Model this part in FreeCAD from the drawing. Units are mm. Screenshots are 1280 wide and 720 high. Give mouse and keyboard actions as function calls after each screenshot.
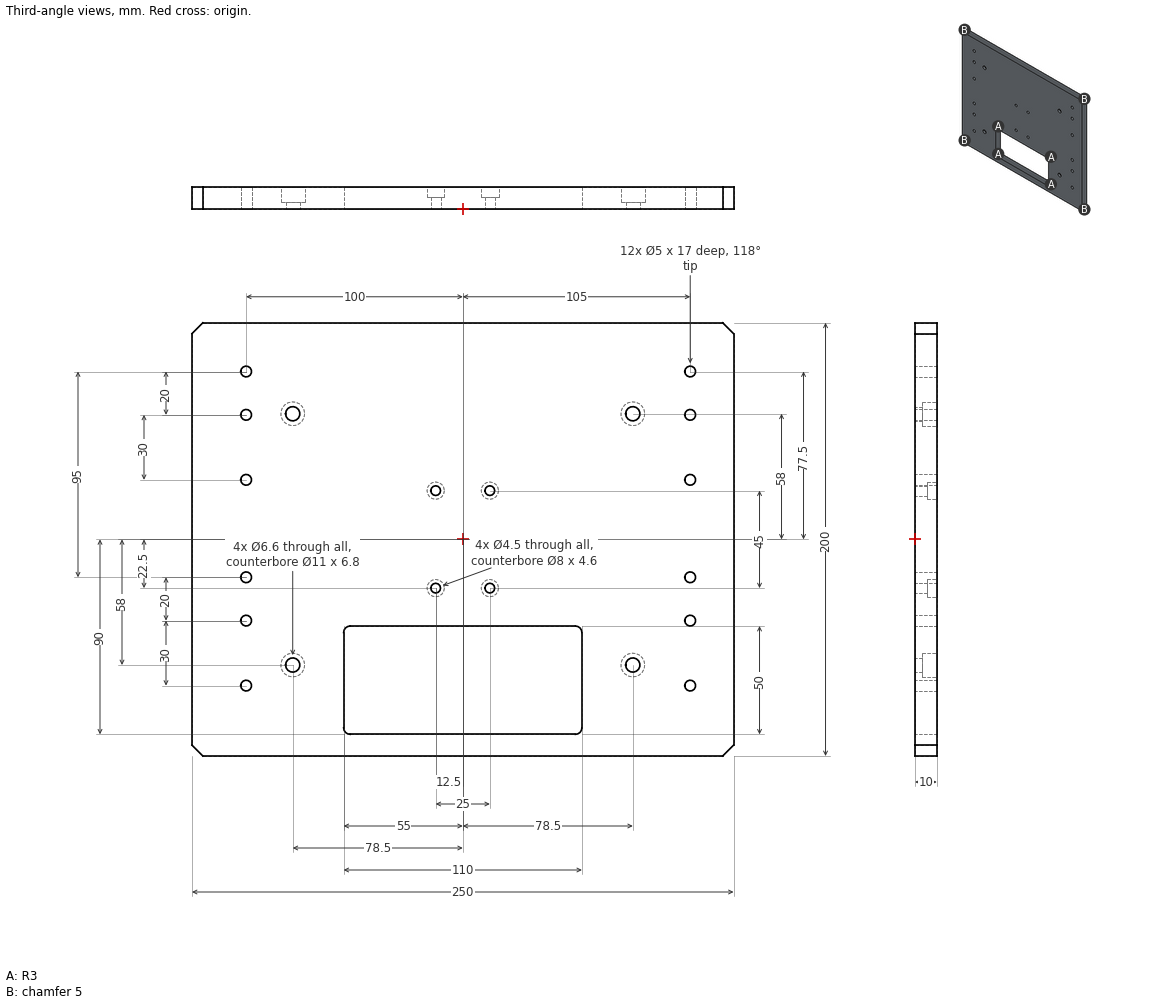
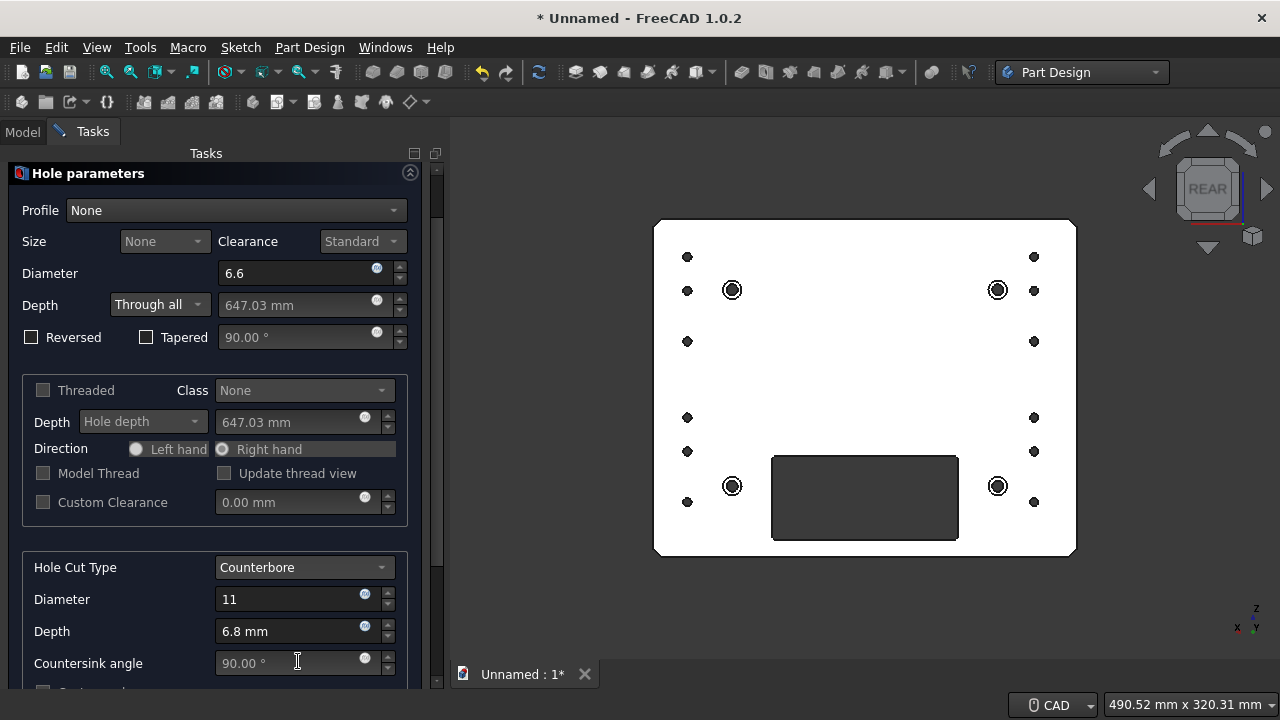
scroll(437, 426, up, 2)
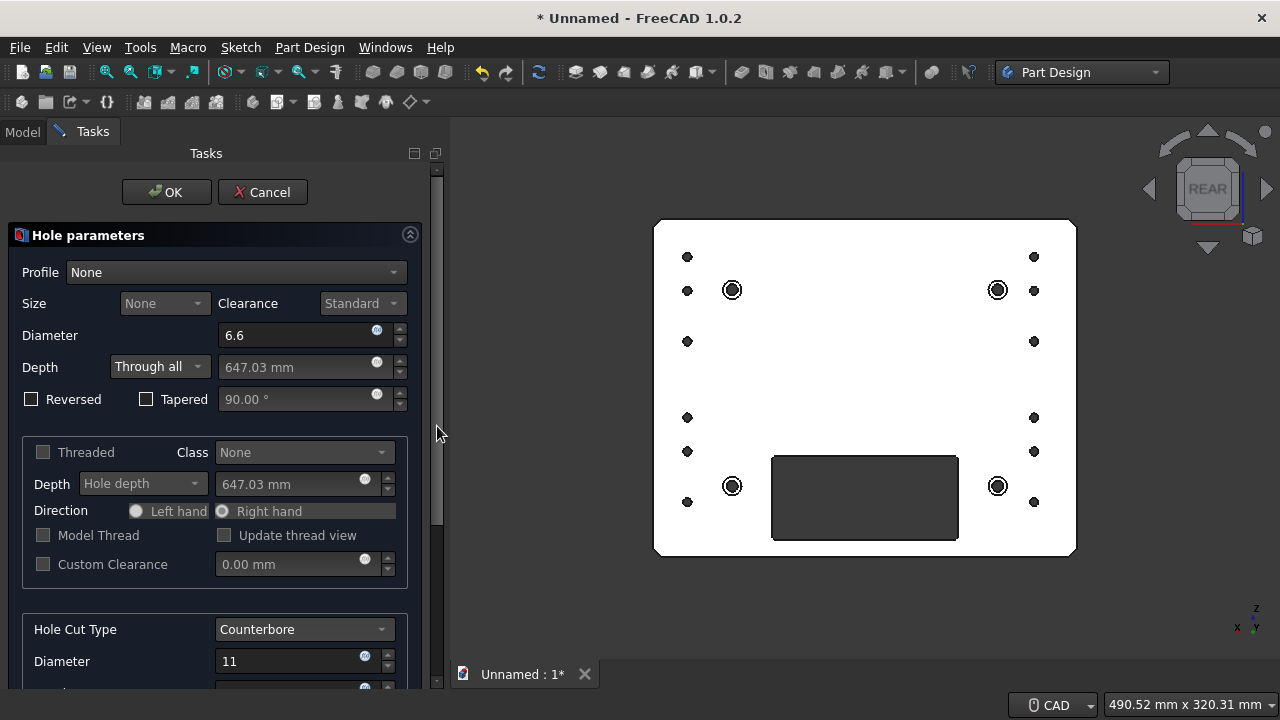
click(167, 192)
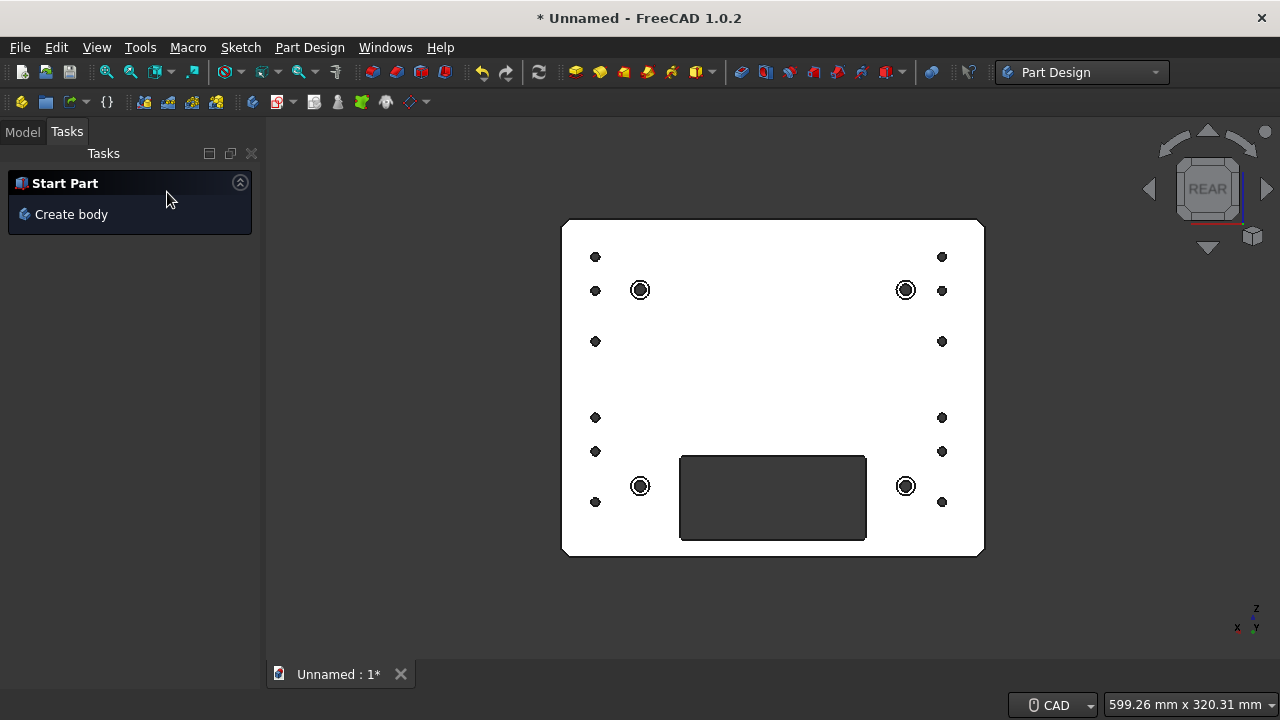
click(773, 339)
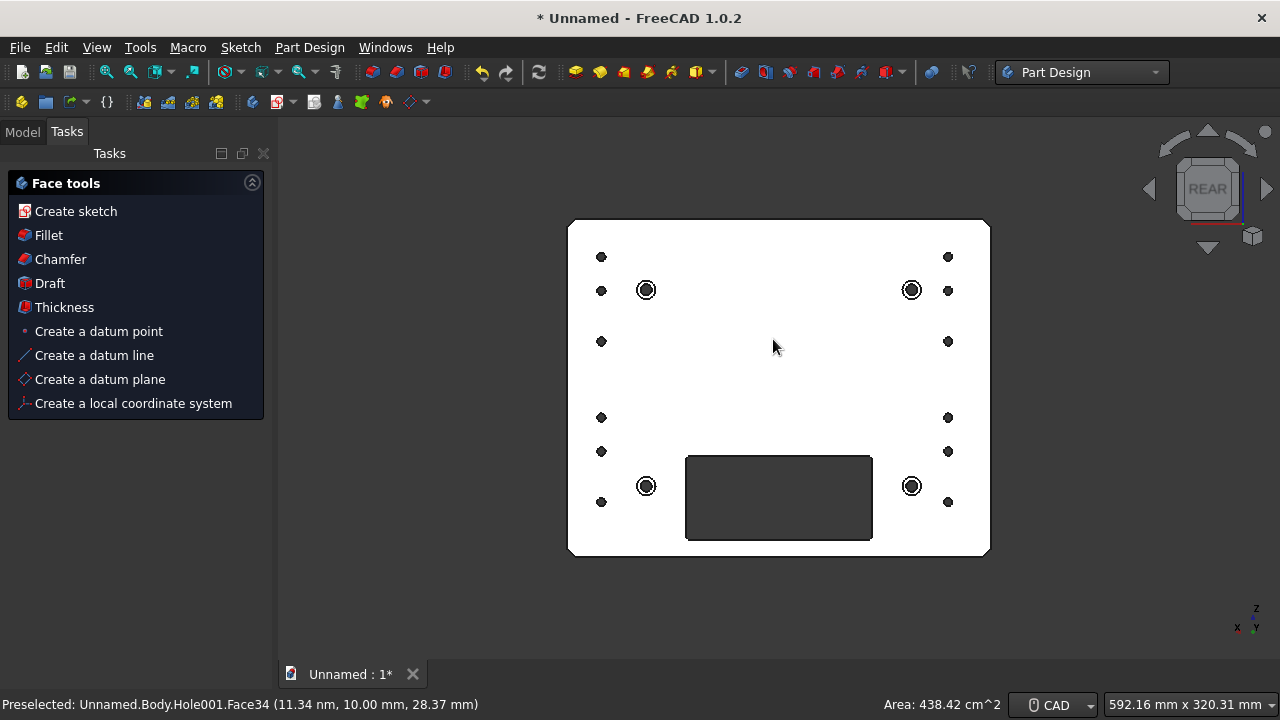
click(278, 102)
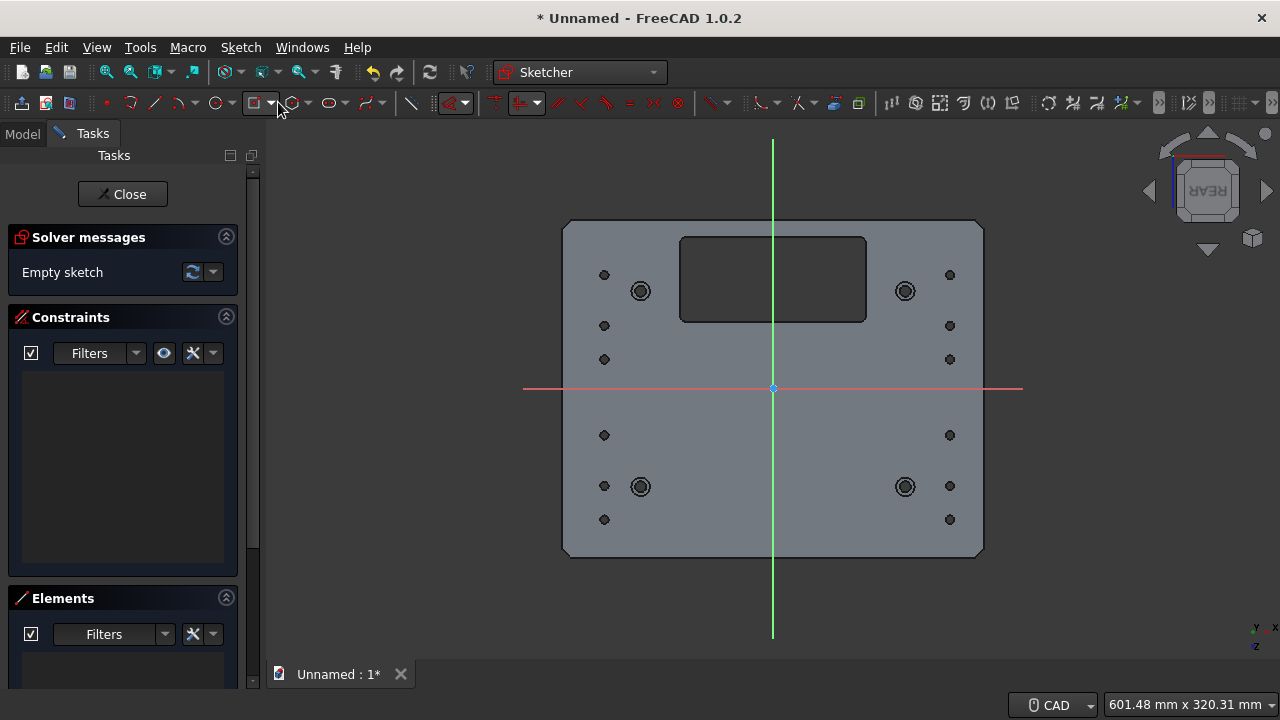
scroll(795, 389, up, 7)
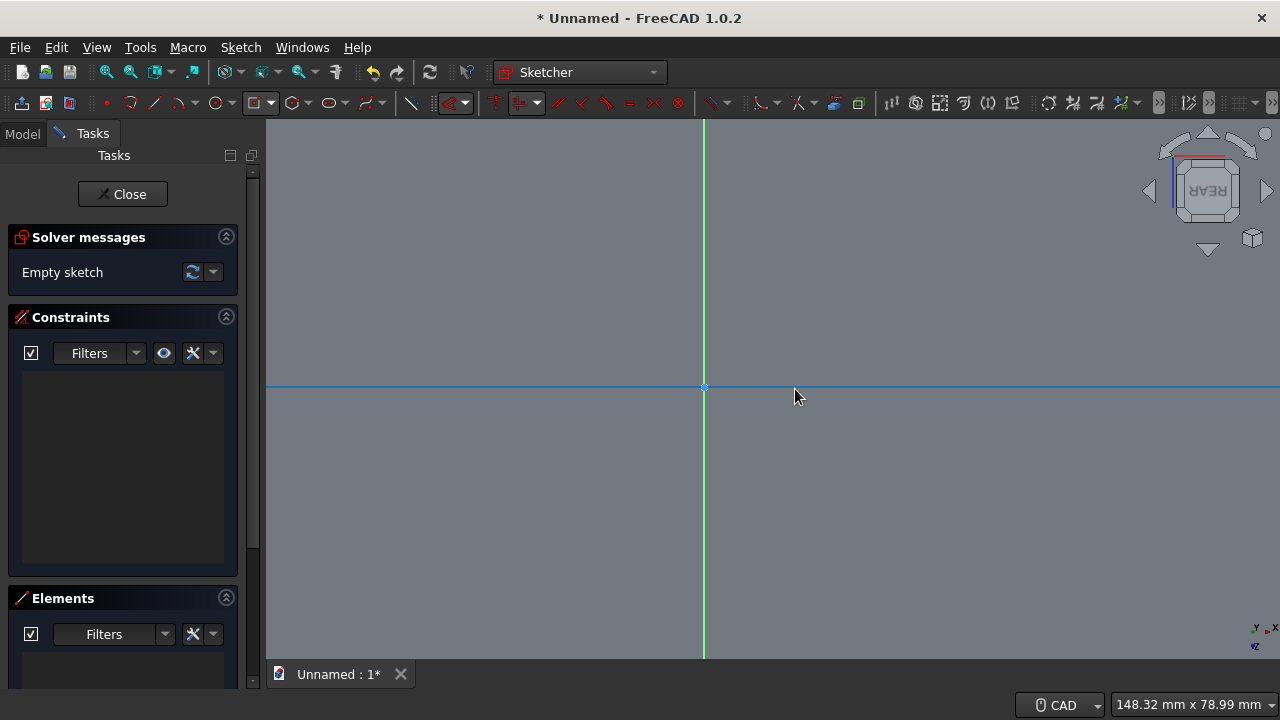
click(216, 104)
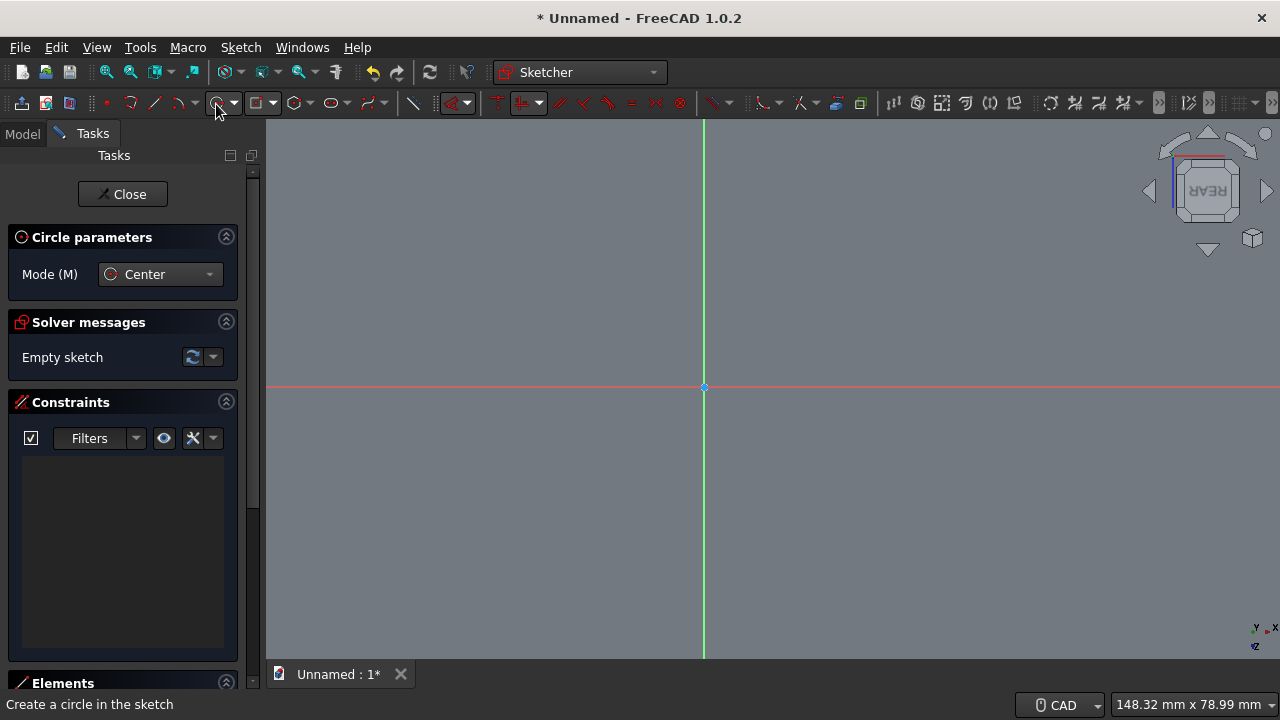
scroll(619, 234, up, 2)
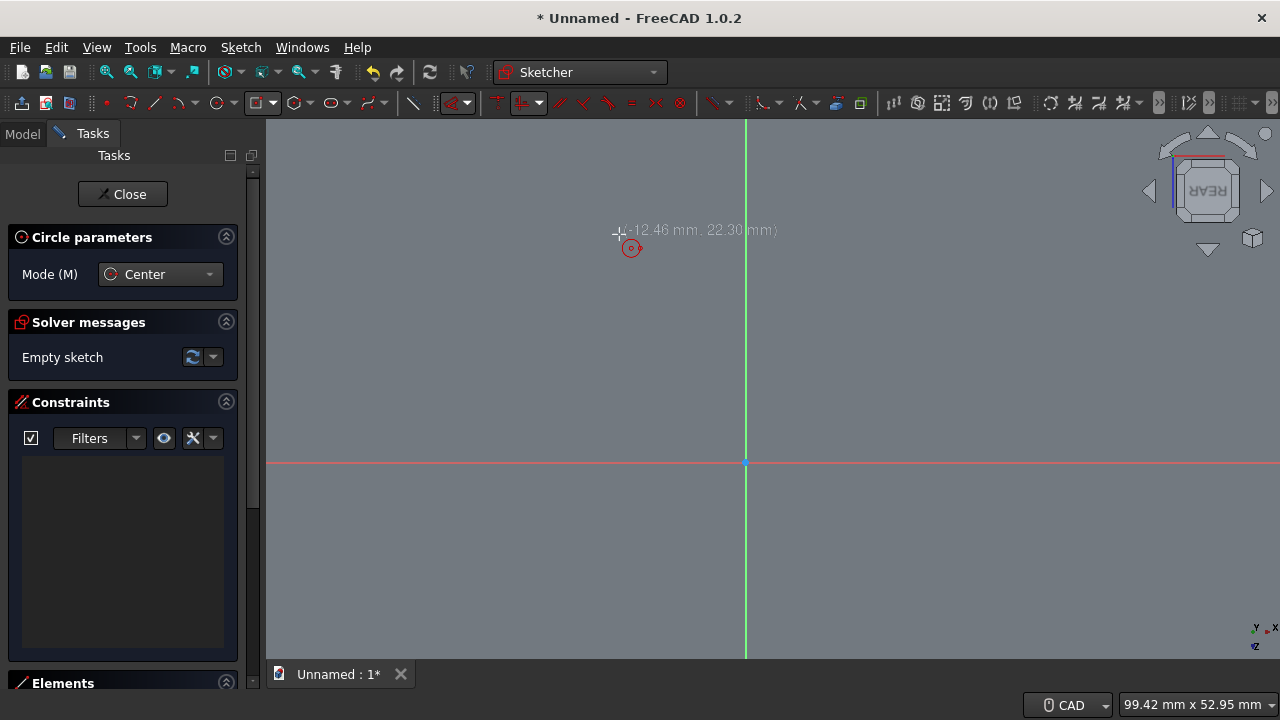
click(618, 233)
move(635, 217)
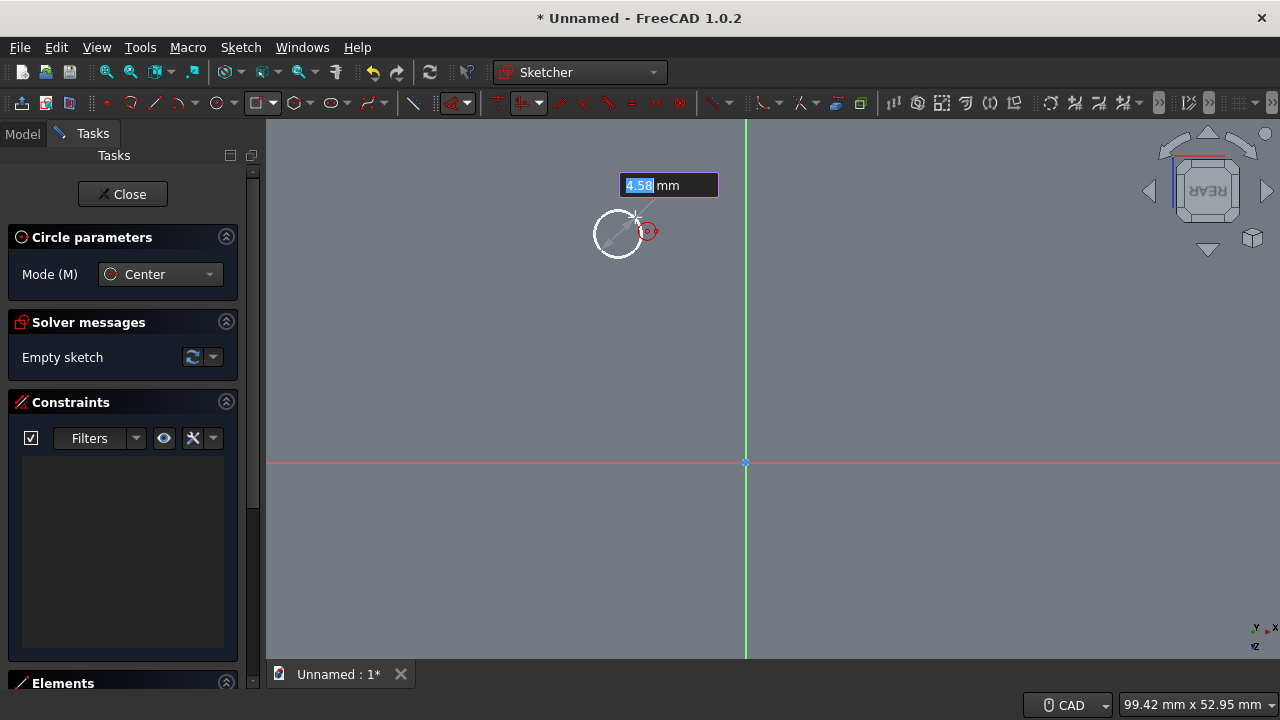
text(4.5)
key(Return)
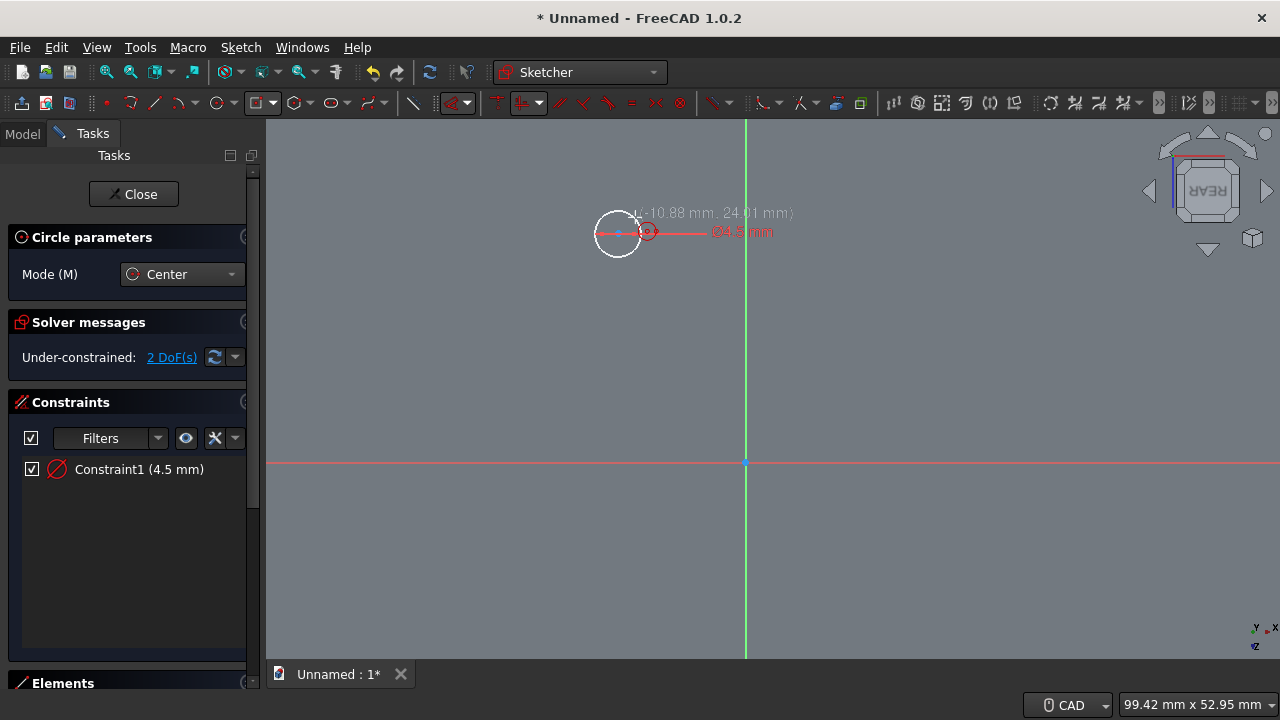
click(873, 233)
move(890, 217)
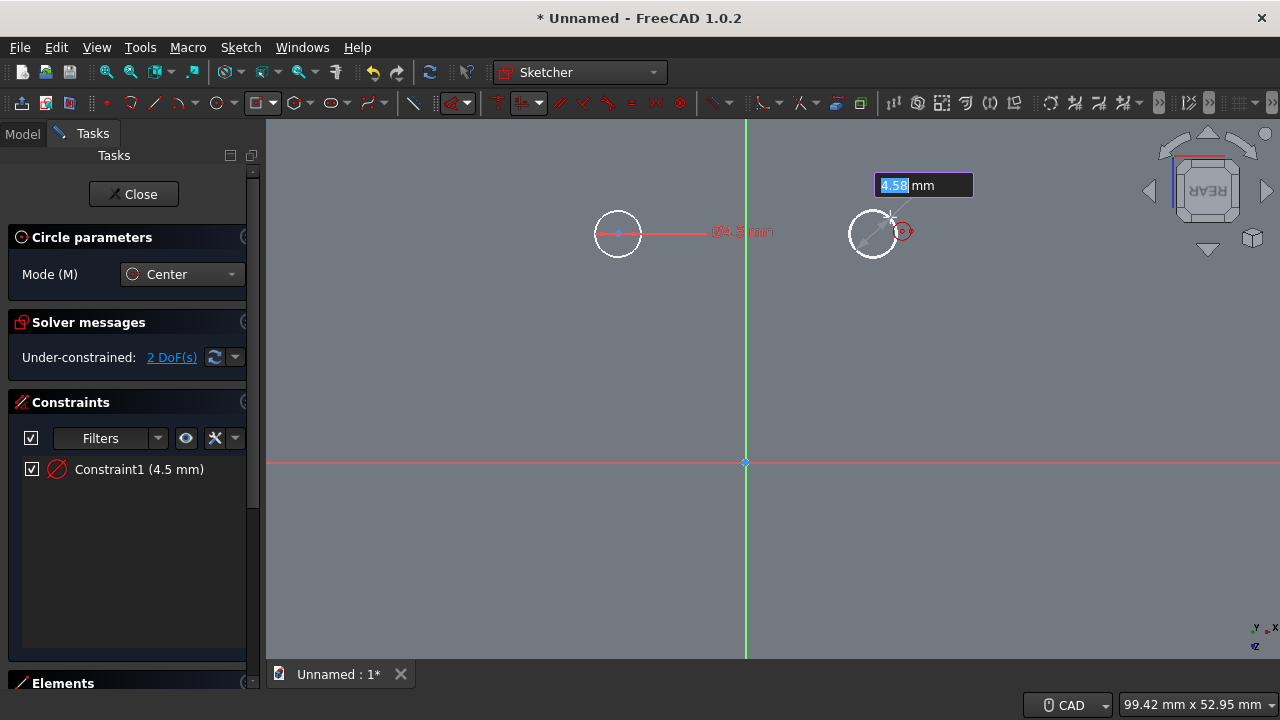
text(4.5)
key(Return)